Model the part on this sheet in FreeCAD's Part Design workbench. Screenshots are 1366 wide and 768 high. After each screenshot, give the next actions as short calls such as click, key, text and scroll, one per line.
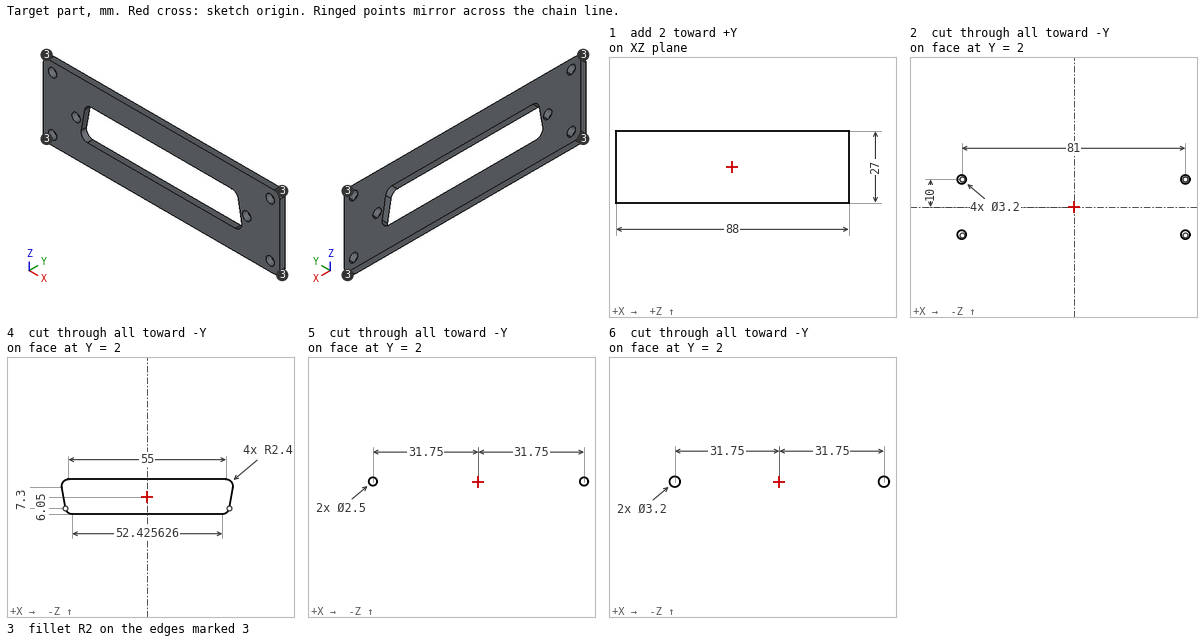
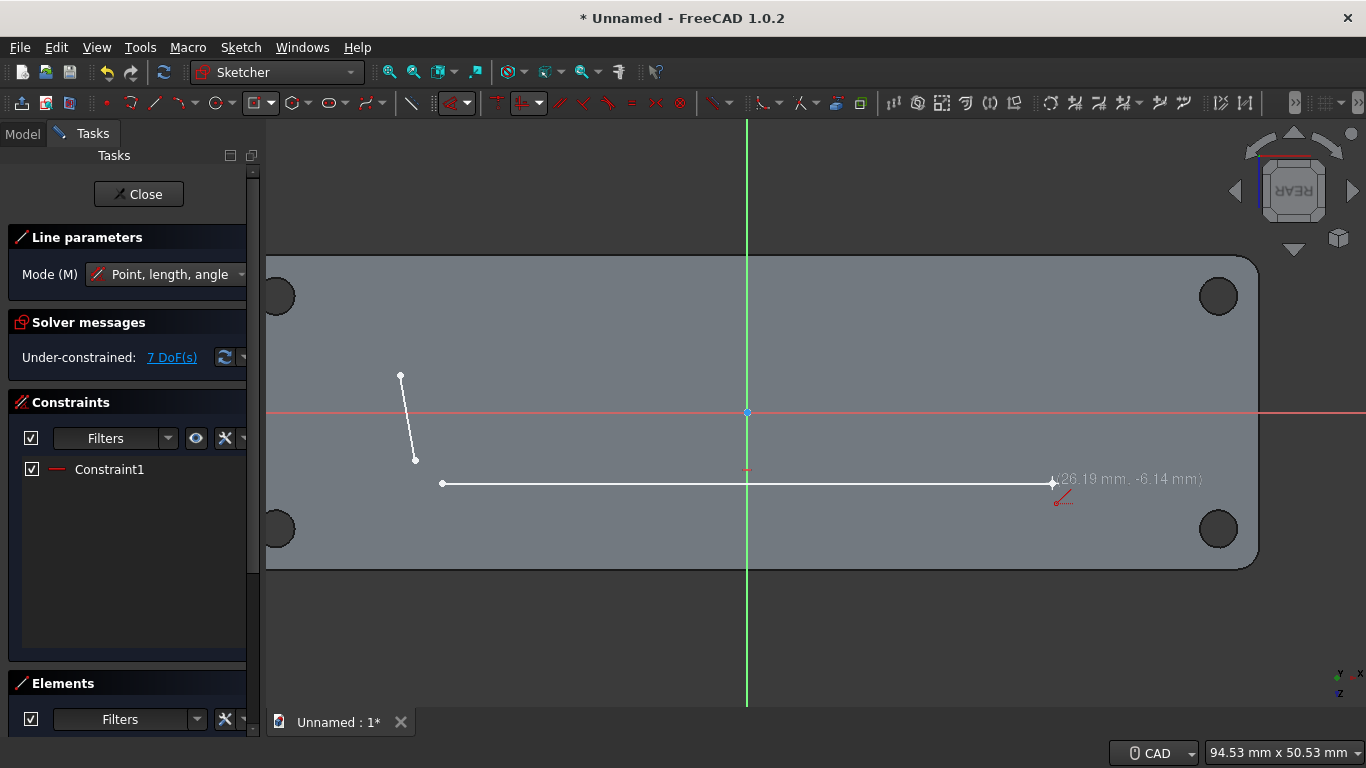
click(1080, 460)
click(1095, 375)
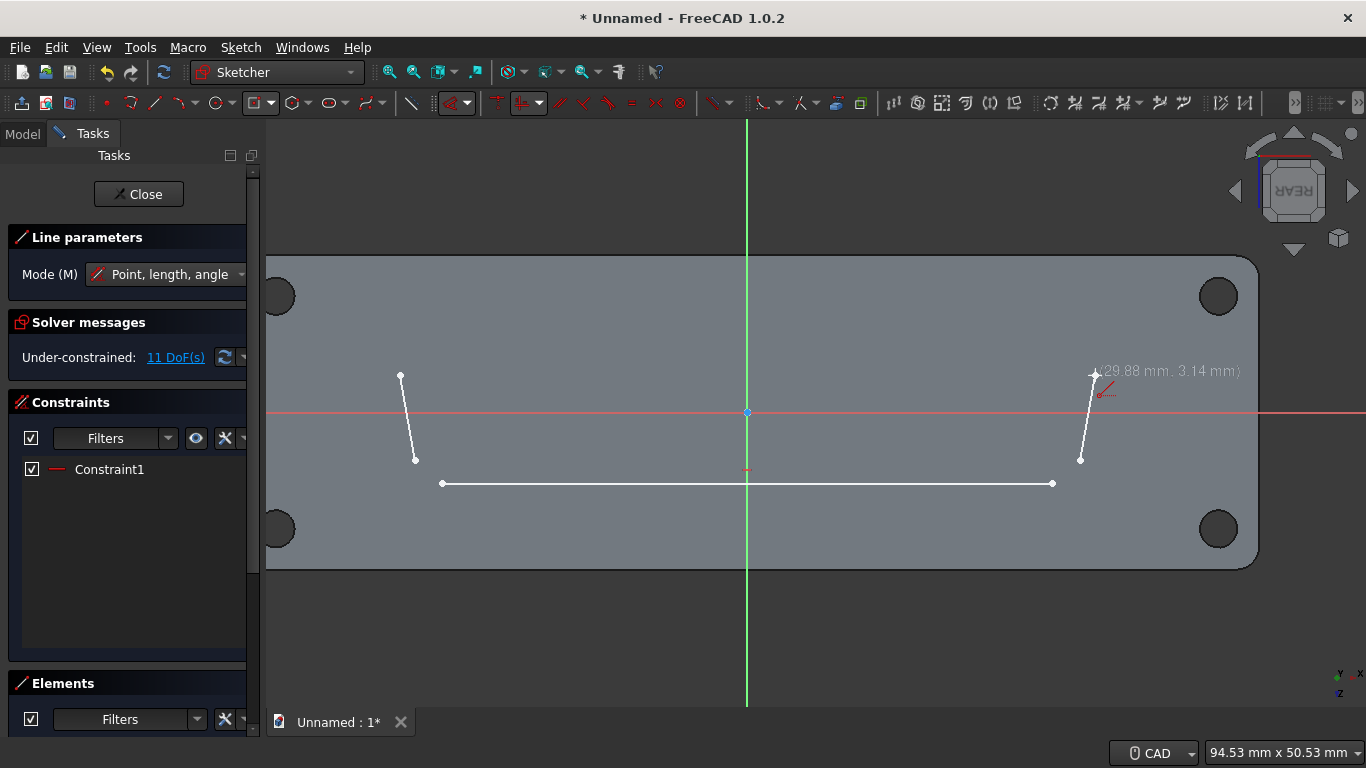
click(1067, 342)
click(427, 342)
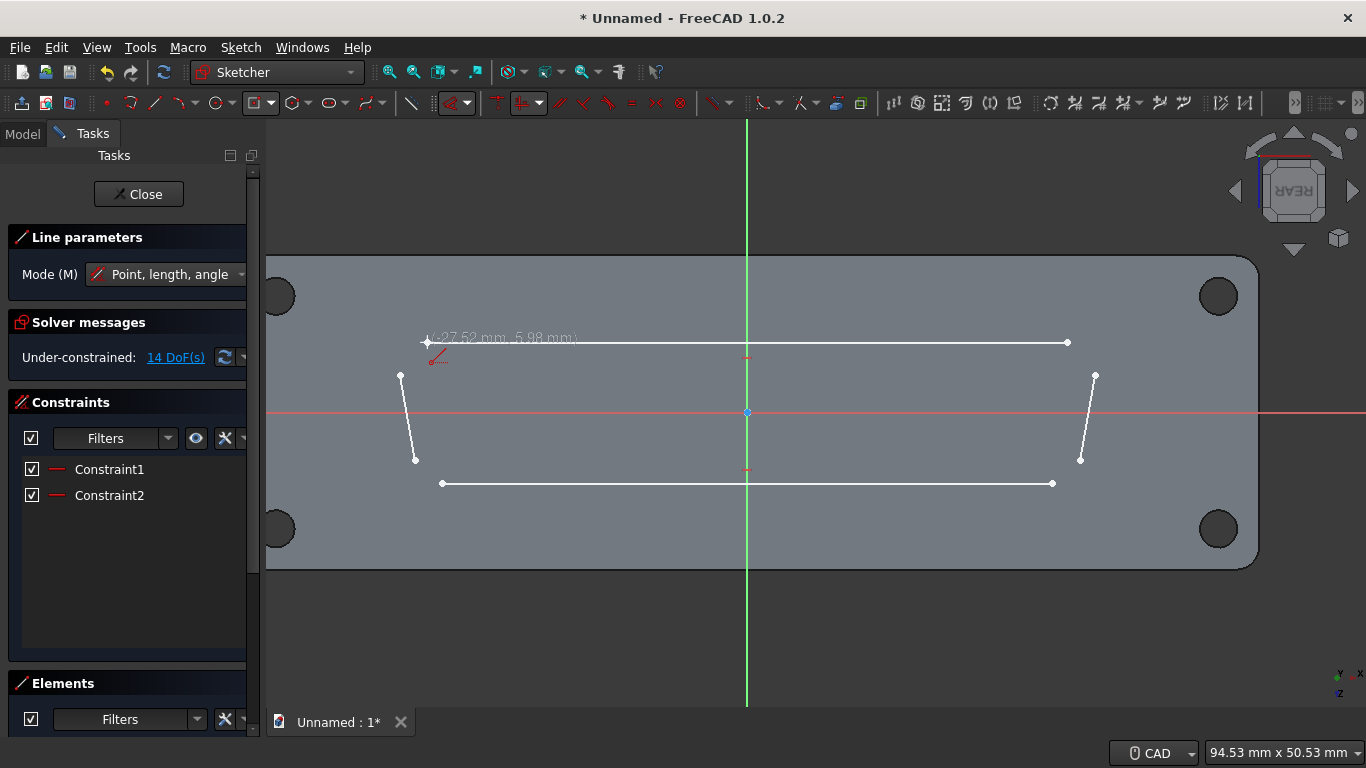
key(g)
key(3)
key(a)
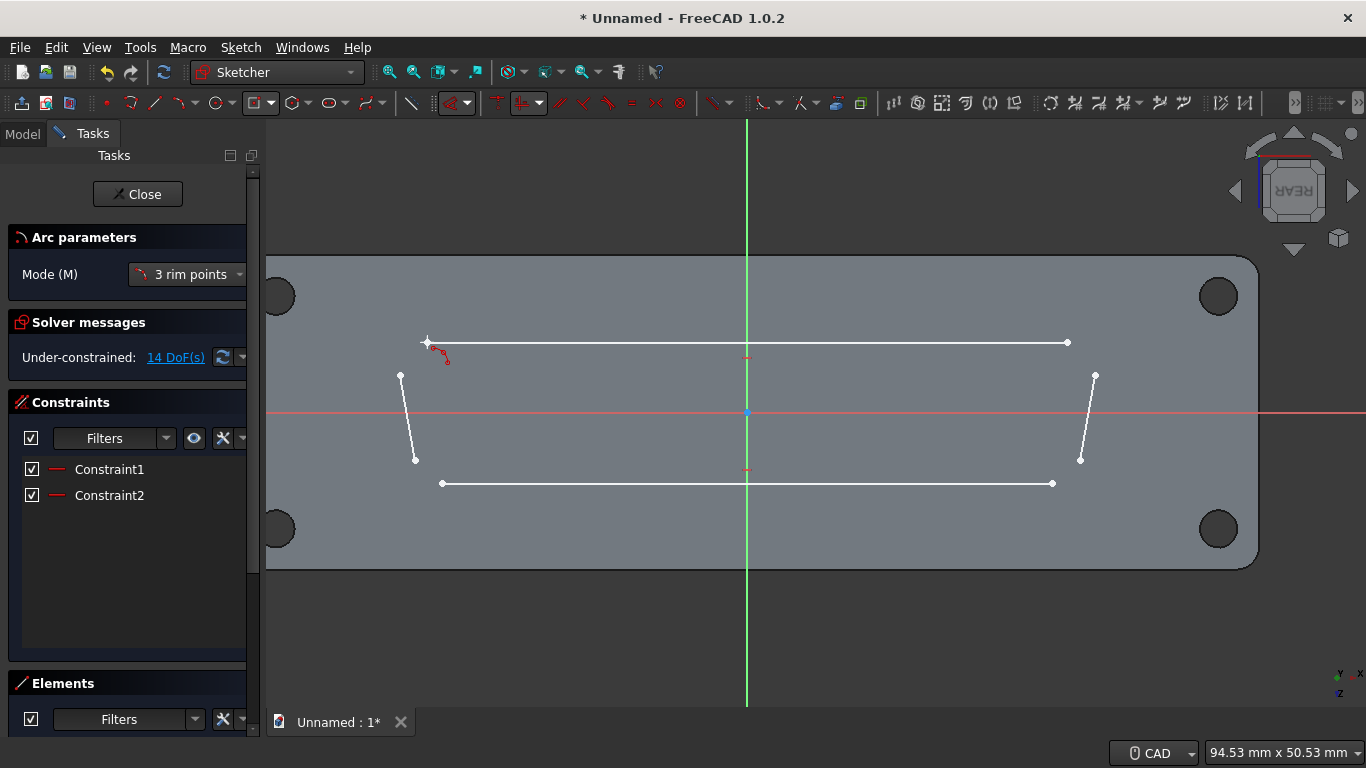
click(415, 461)
click(442, 484)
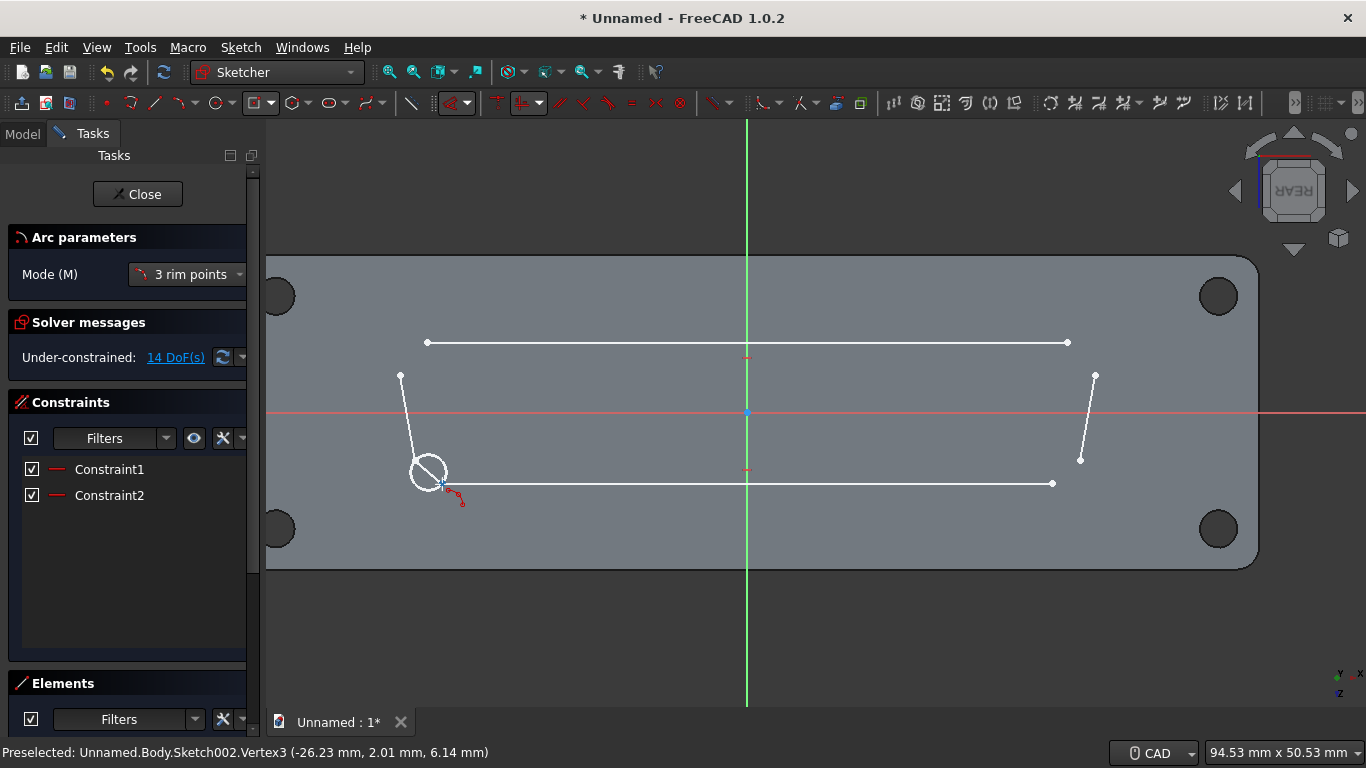
scroll(424, 476, up, 5)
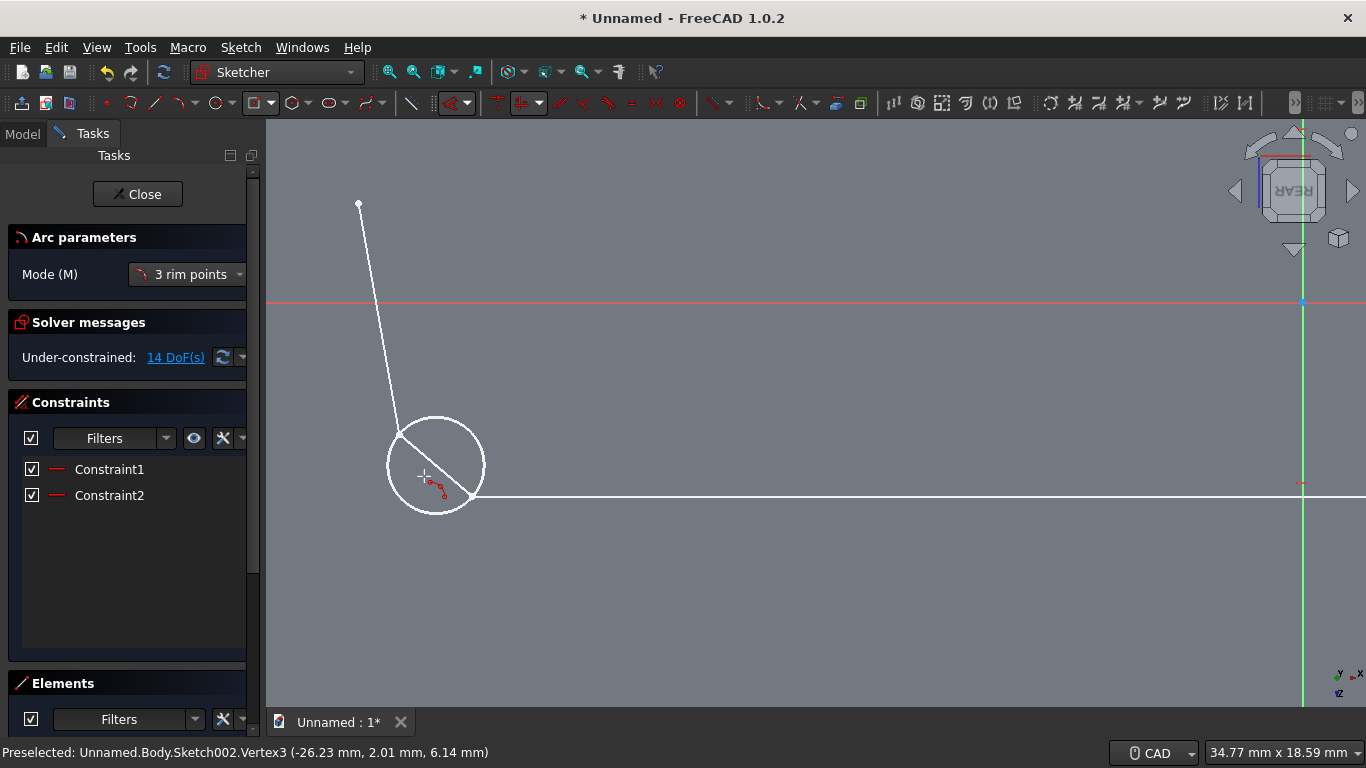
click(425, 476)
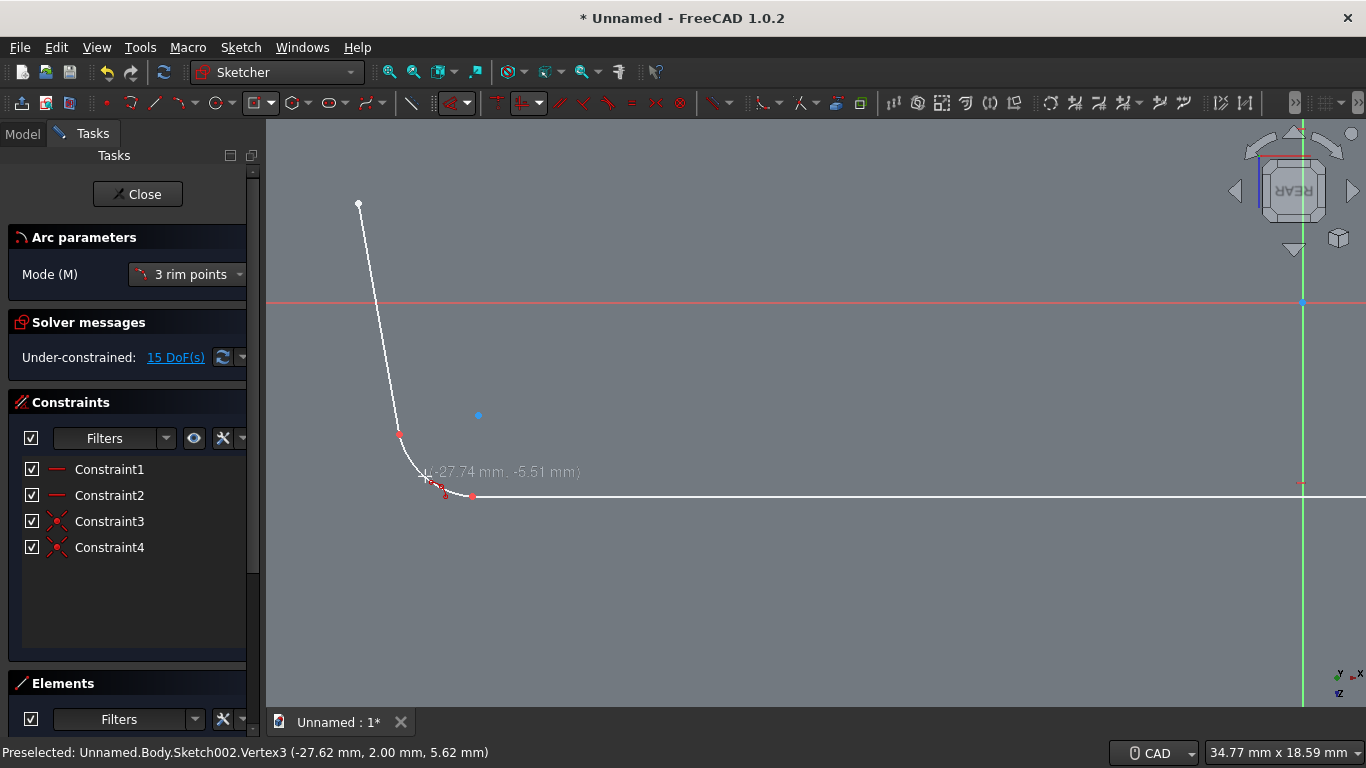
scroll(424, 477, down, 5)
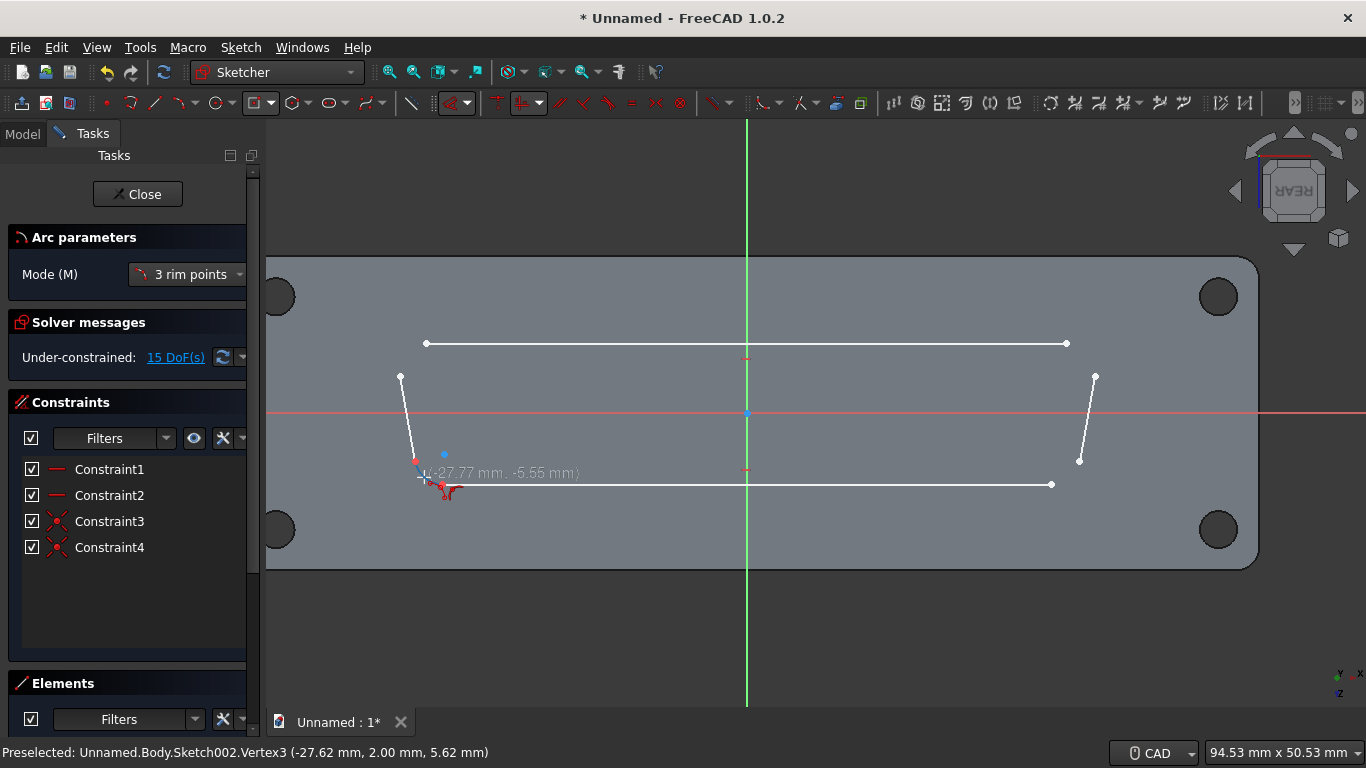
click(1052, 485)
click(1080, 462)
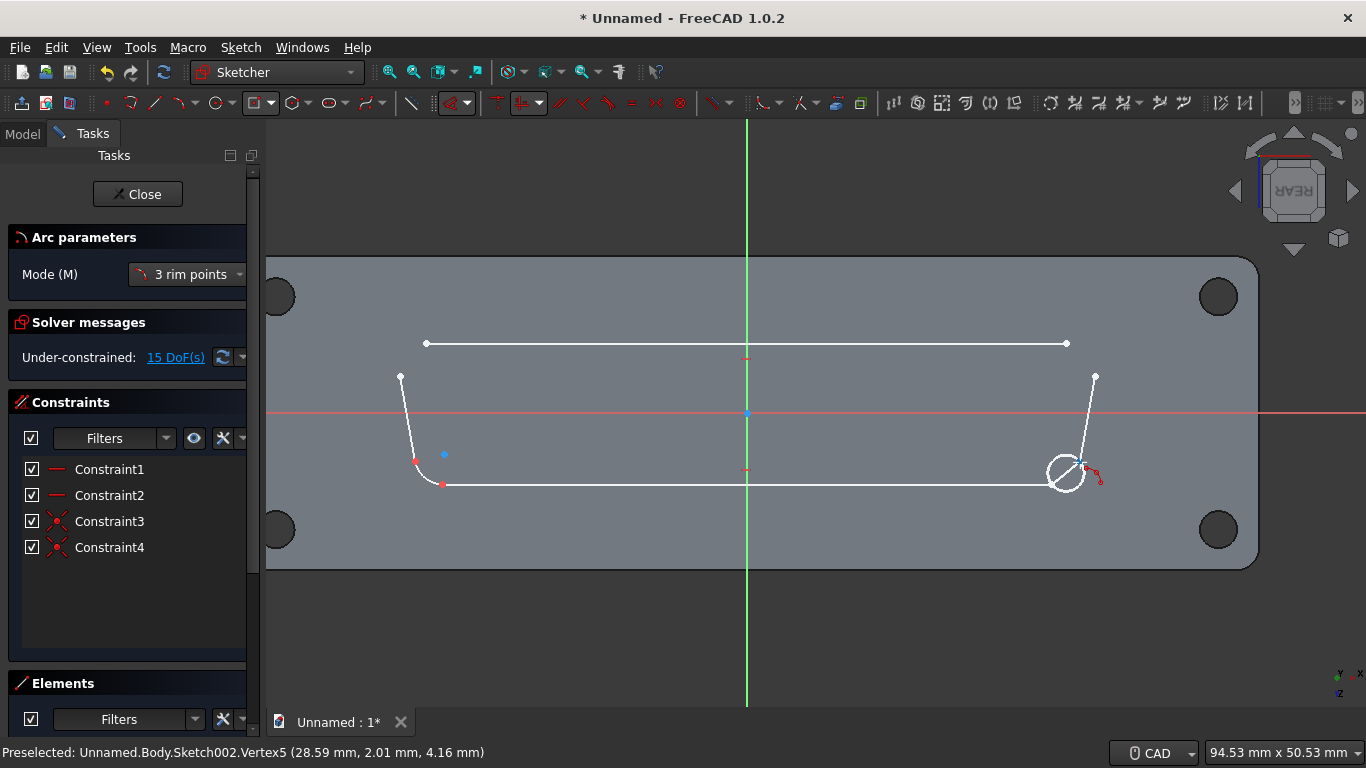
scroll(1070, 477, up, 5)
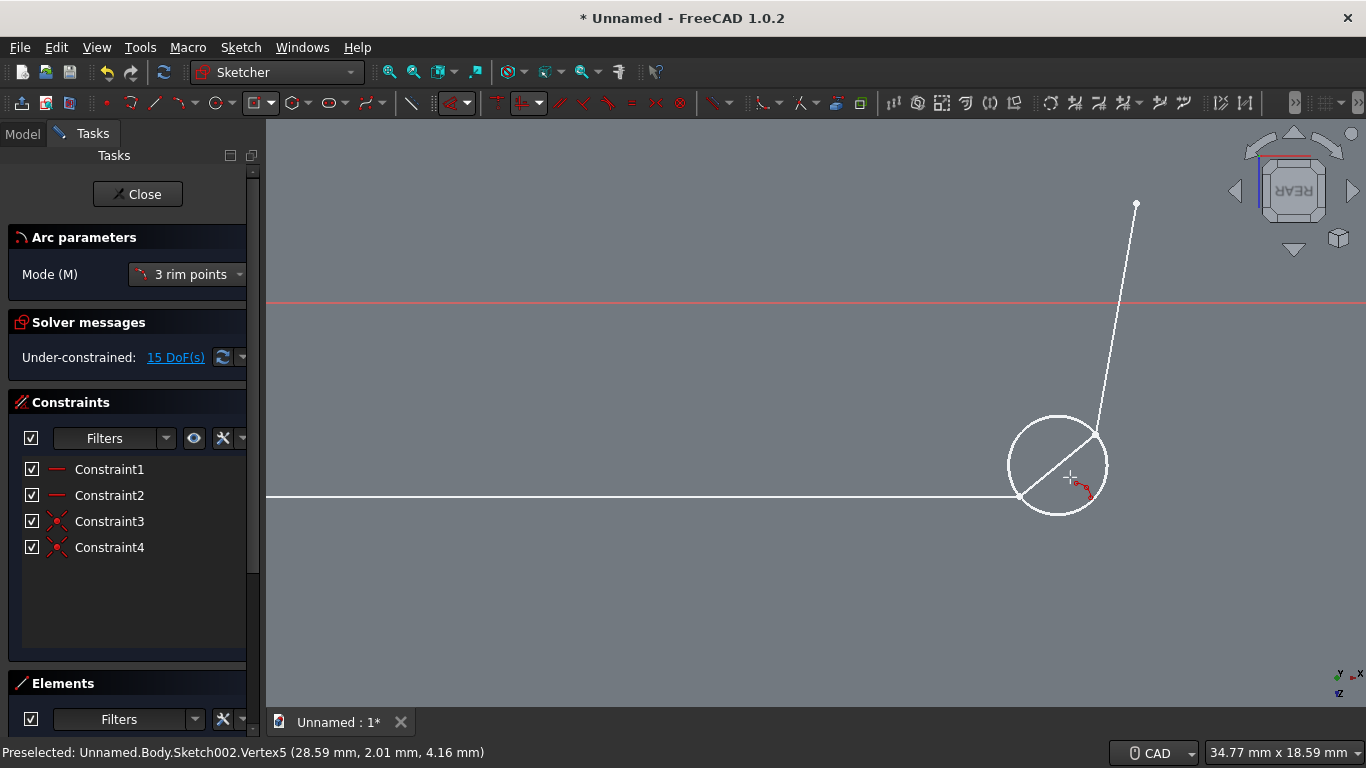
click(1069, 476)